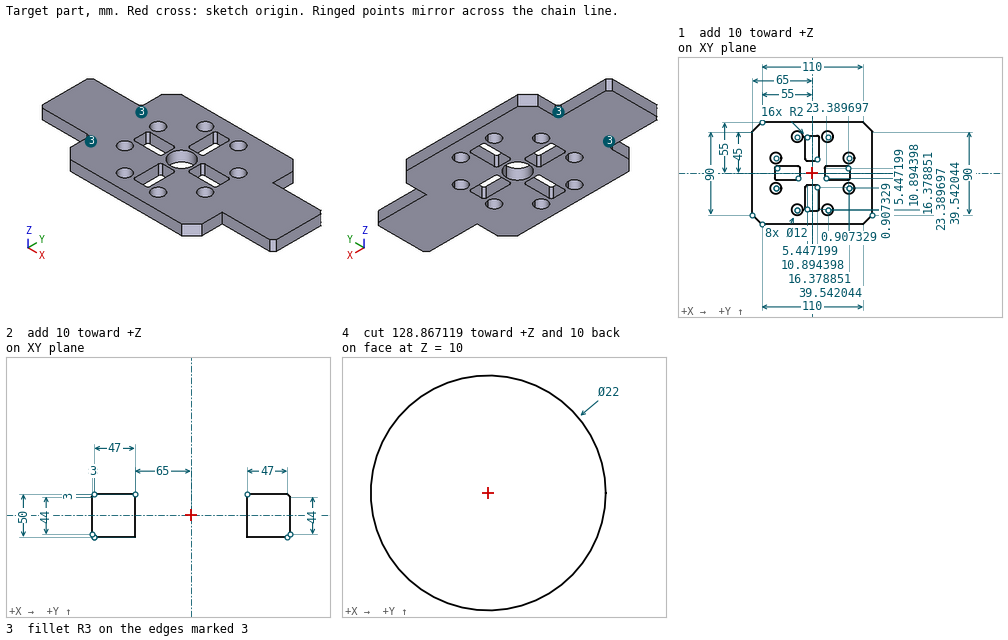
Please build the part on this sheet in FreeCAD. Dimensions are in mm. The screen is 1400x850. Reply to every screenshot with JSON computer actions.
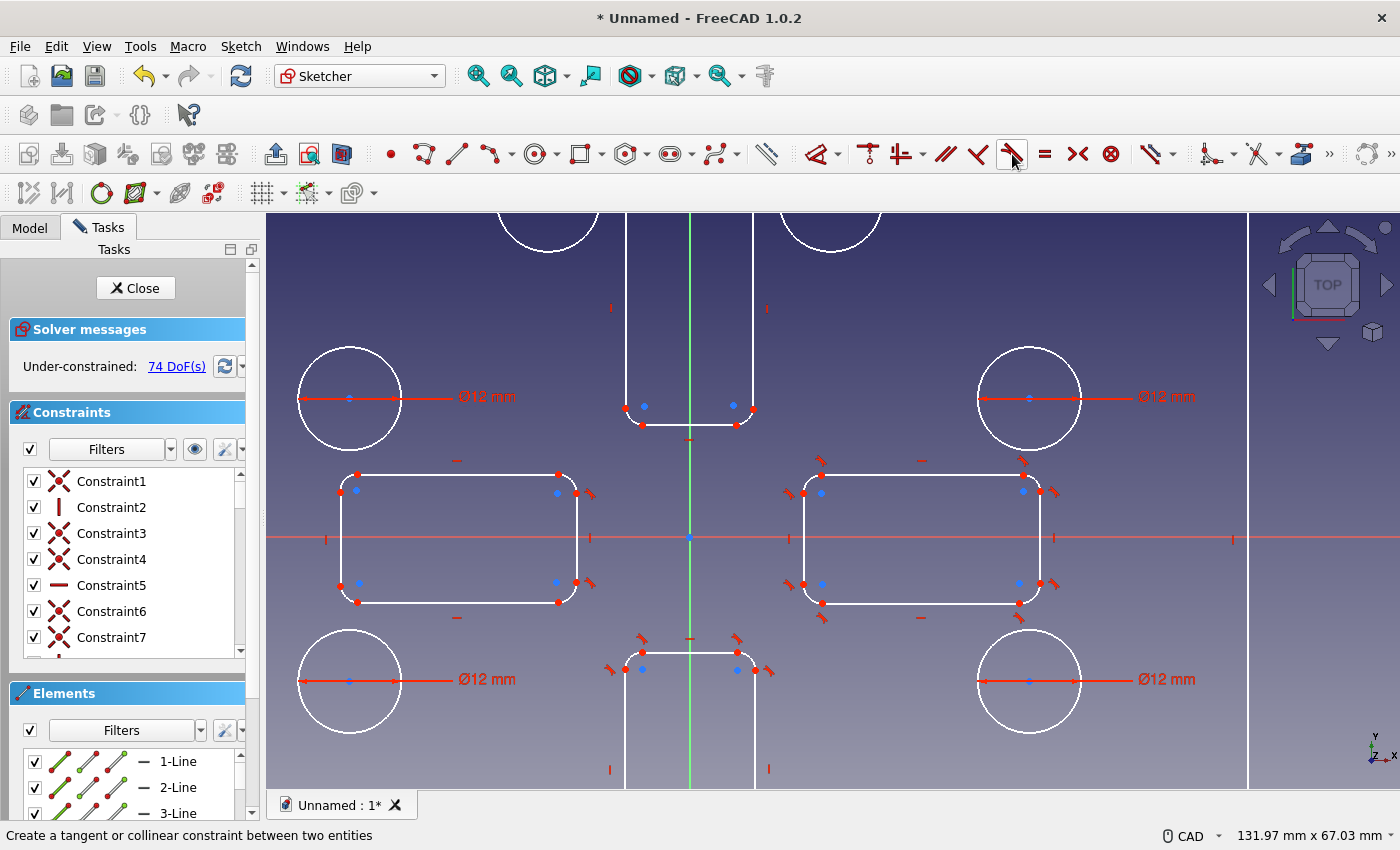
{"action": "left_click", "coordinate": [498, 603]}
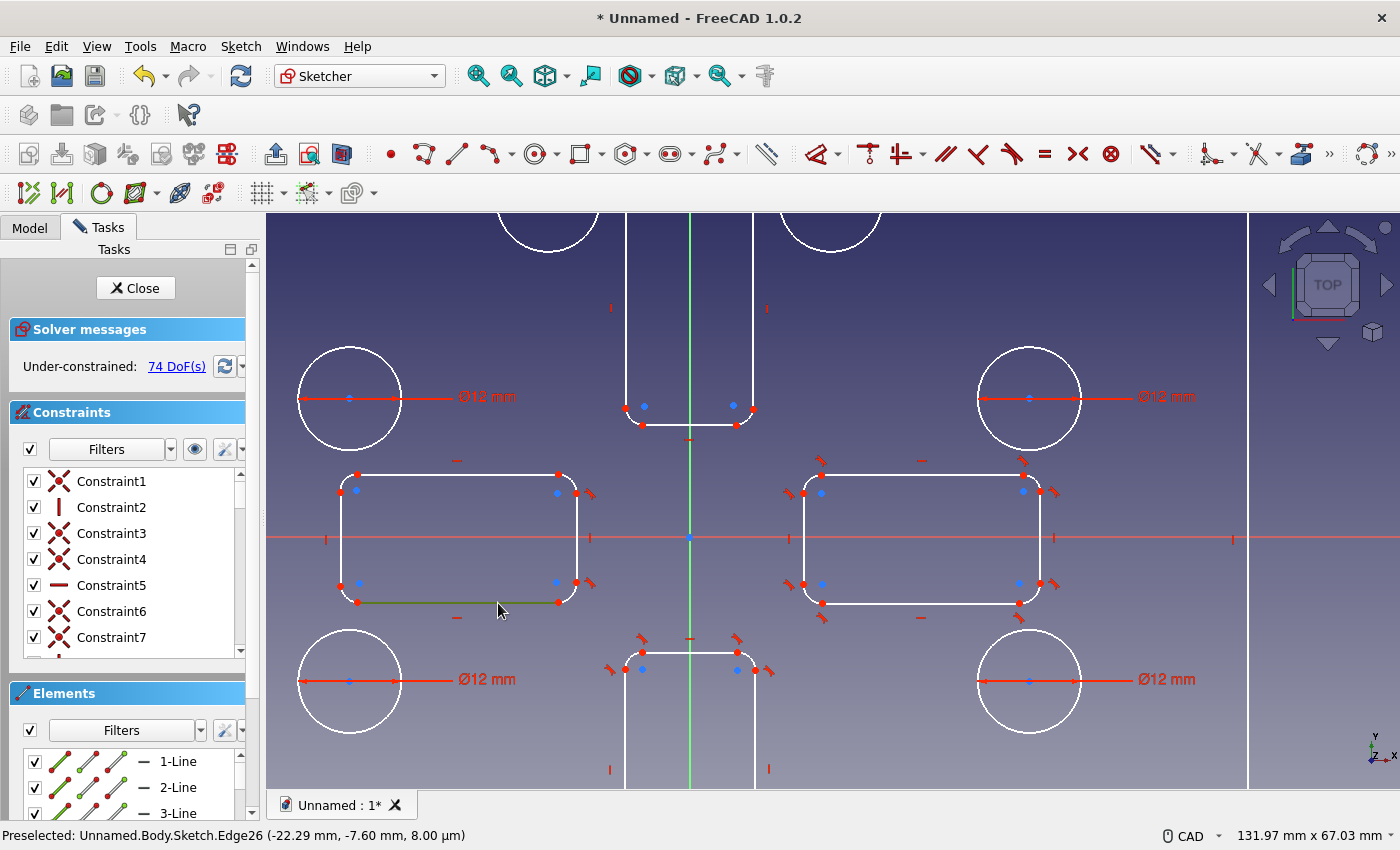
{"action": "left_click", "coordinate": [571, 596]}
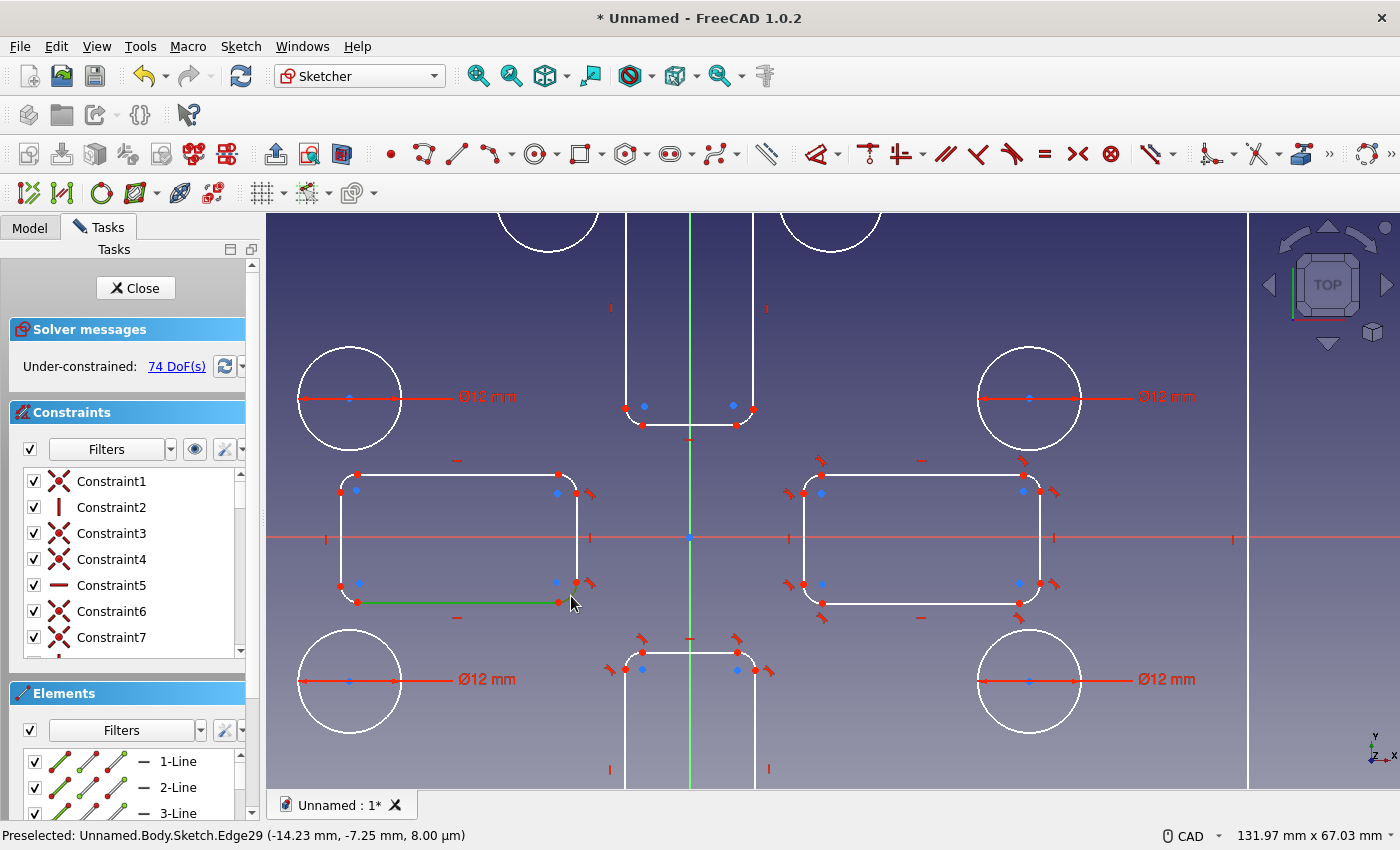
{"action": "left_click", "coordinate": [1012, 154]}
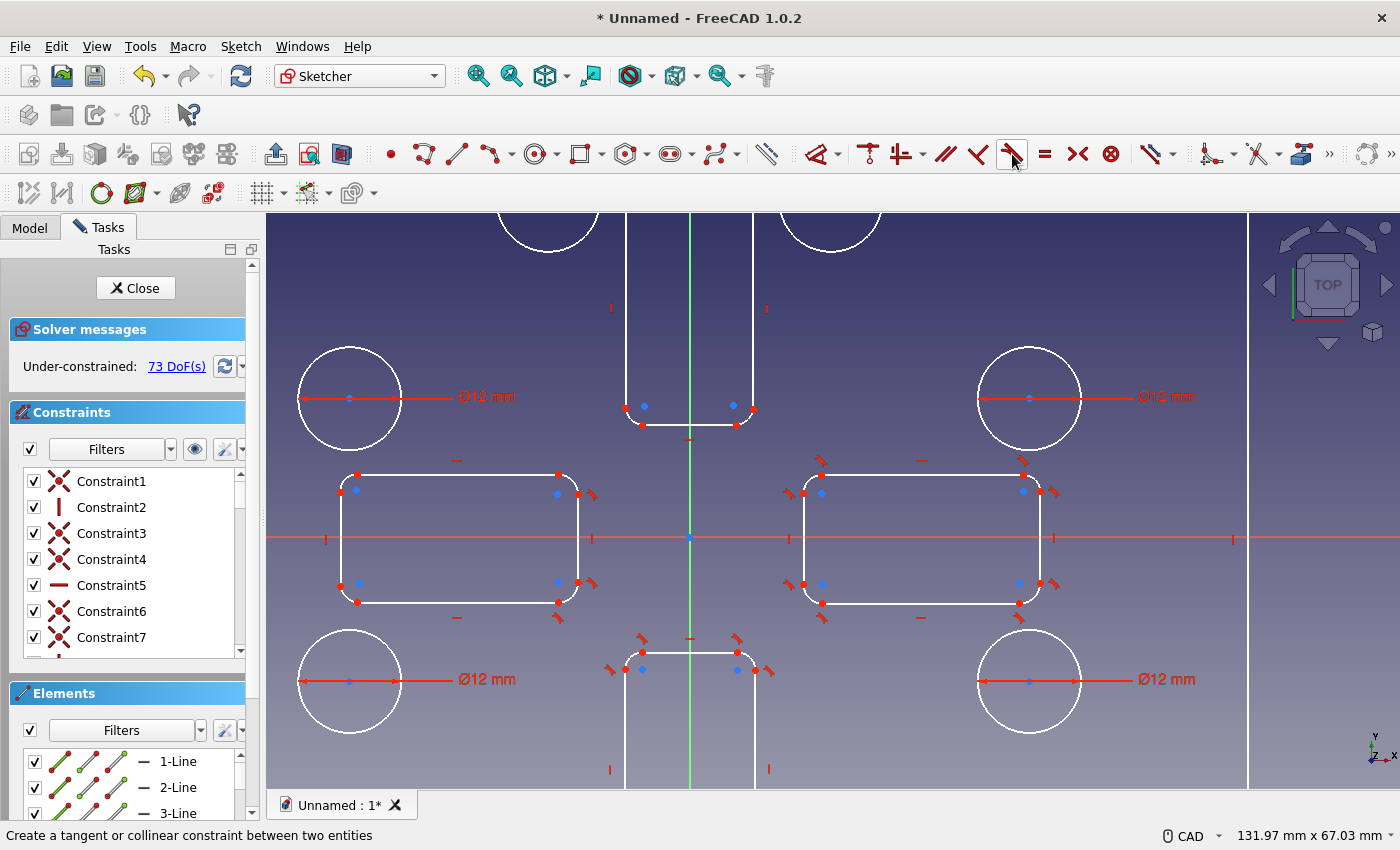
{"action": "left_click", "coordinate": [498, 603]}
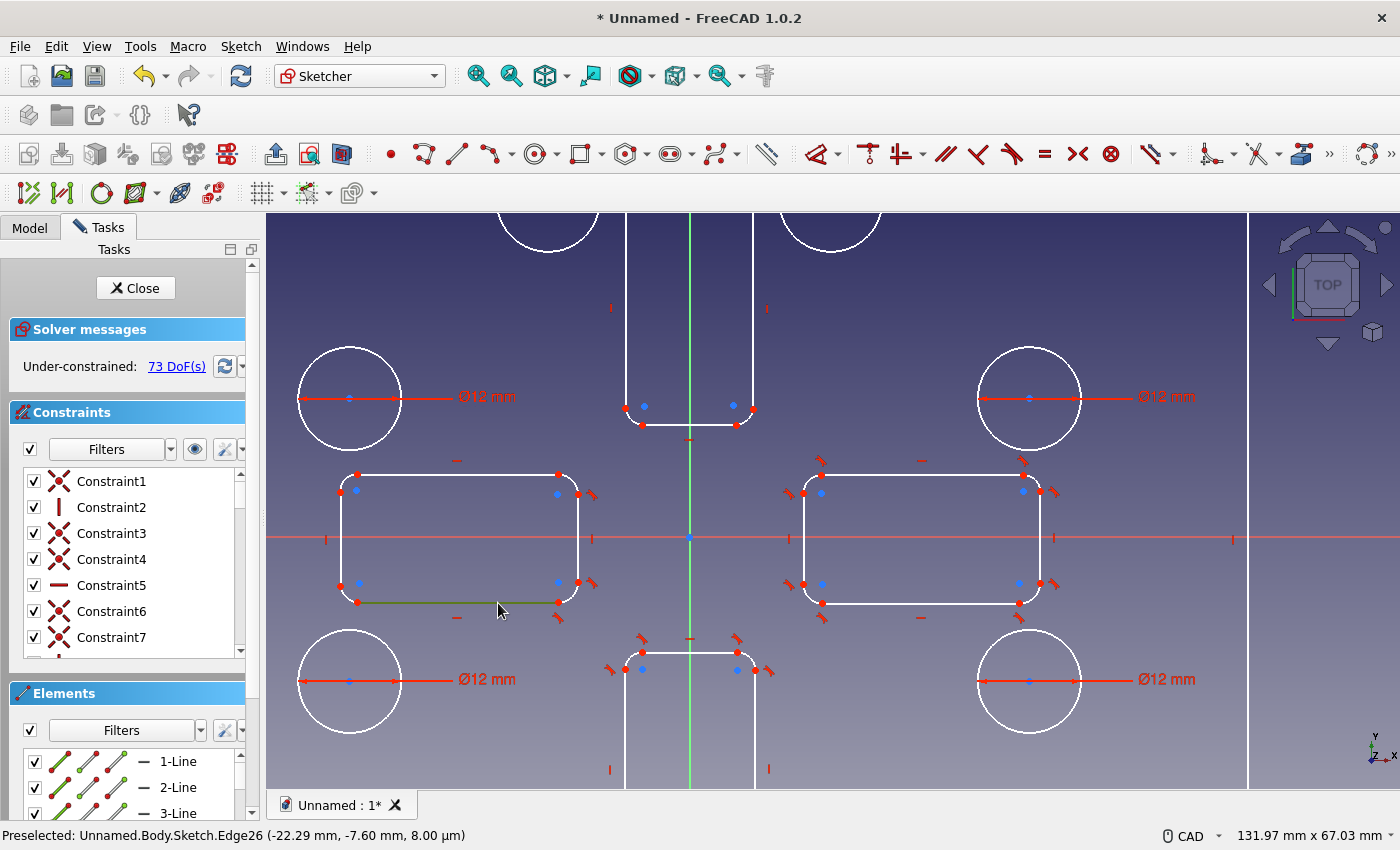
{"action": "left_click", "coordinate": [346, 597]}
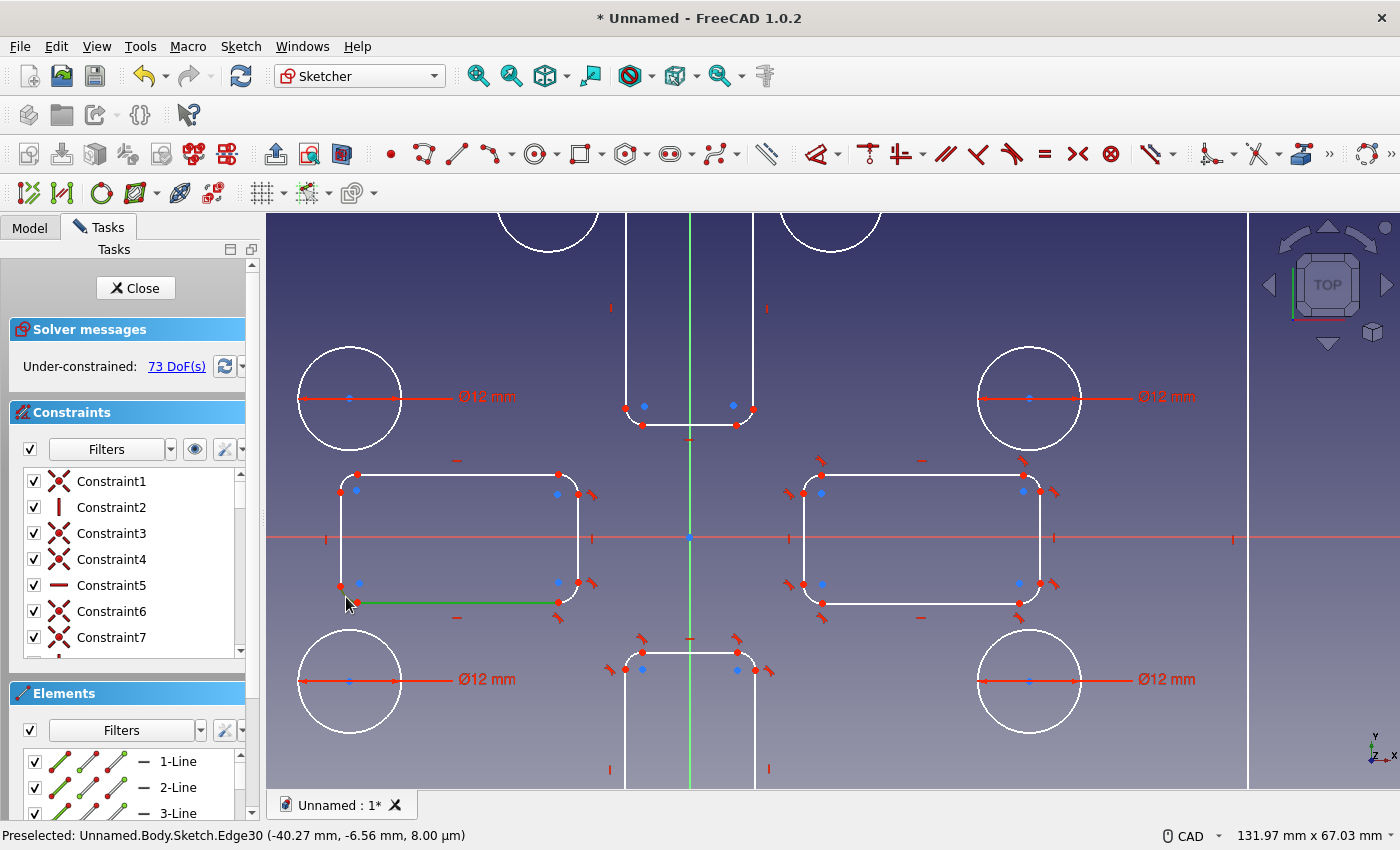
{"action": "left_click", "coordinate": [1012, 154]}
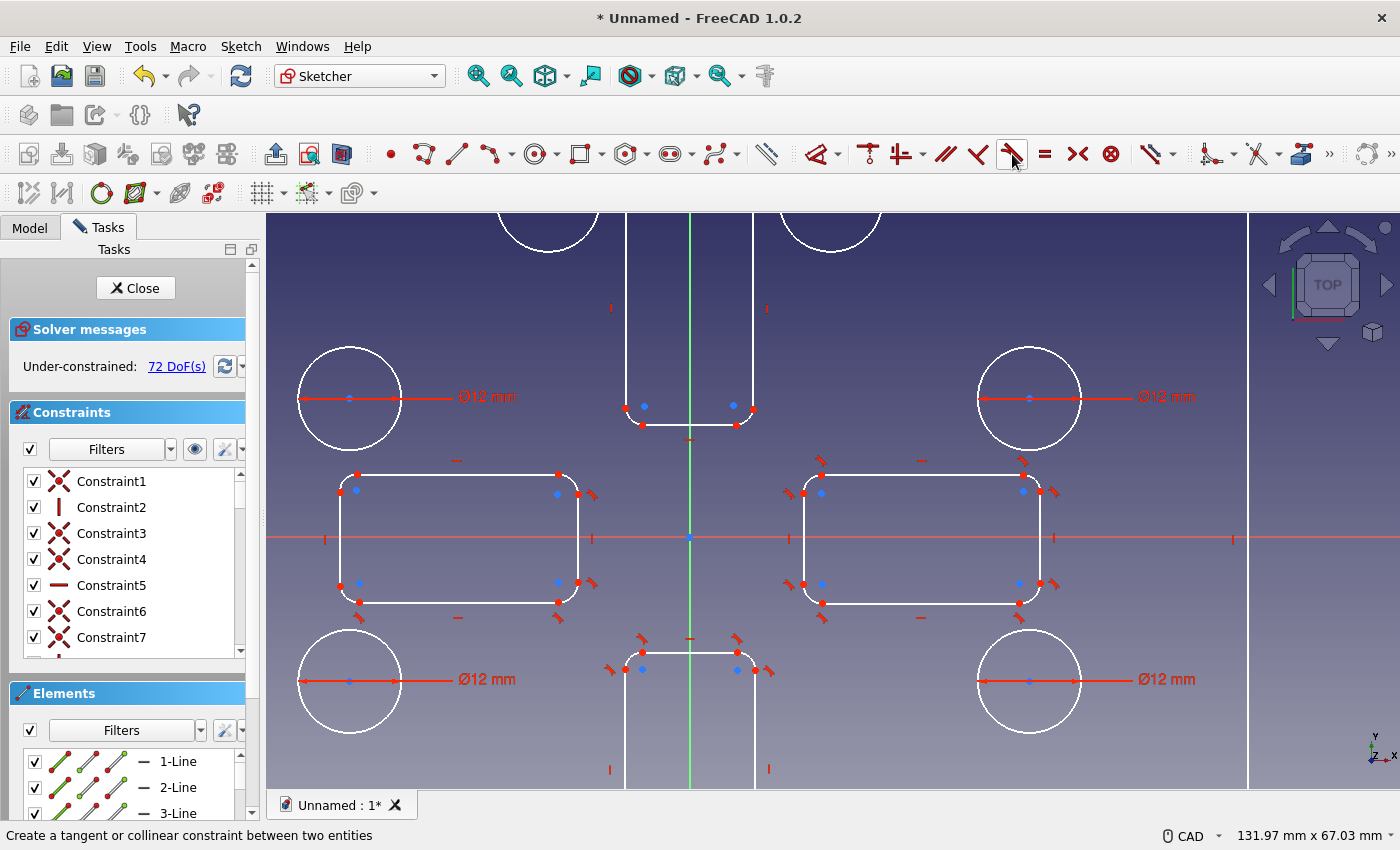
{"action": "left_click", "coordinate": [340, 558]}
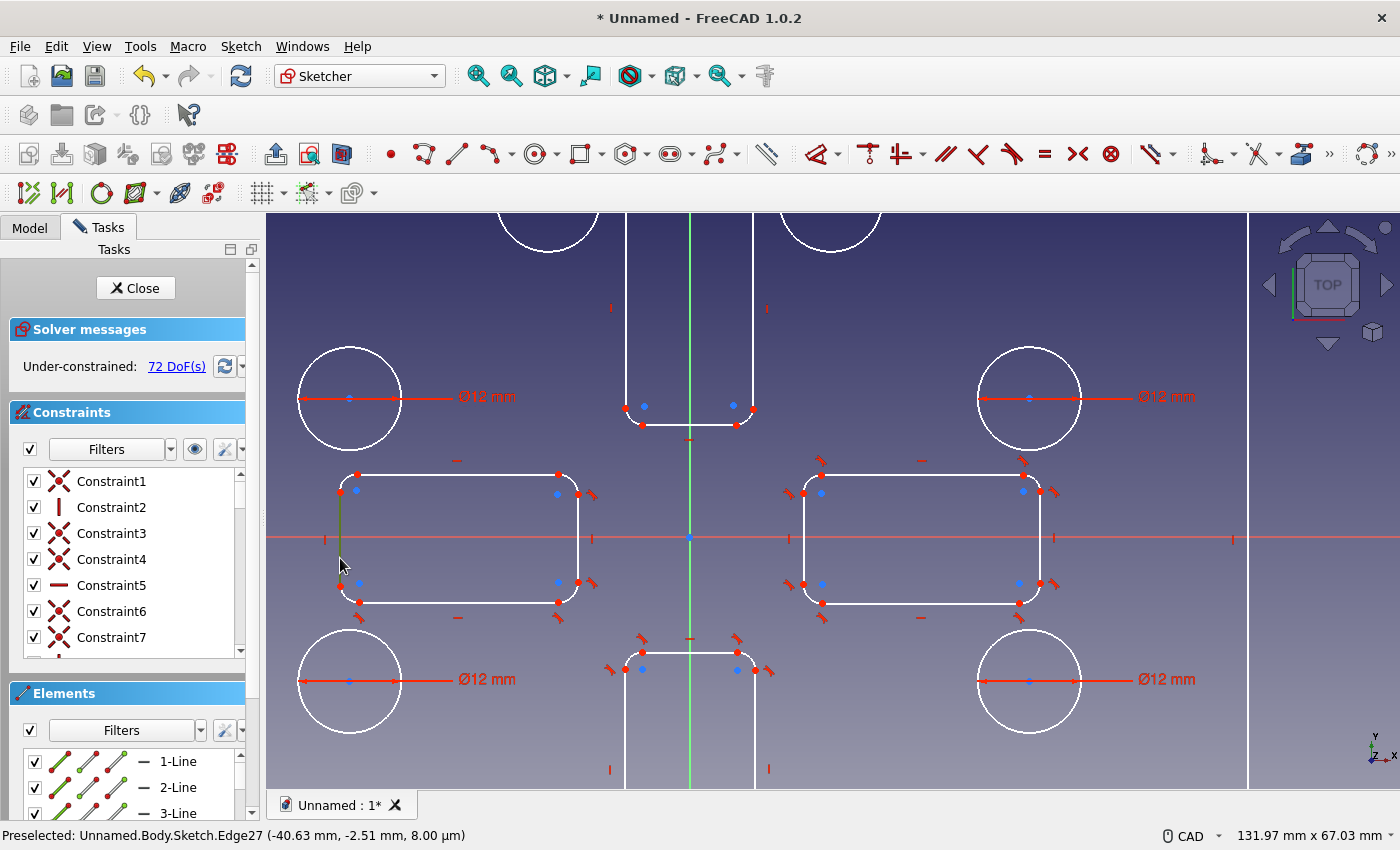
{"action": "left_click", "coordinate": [347, 598]}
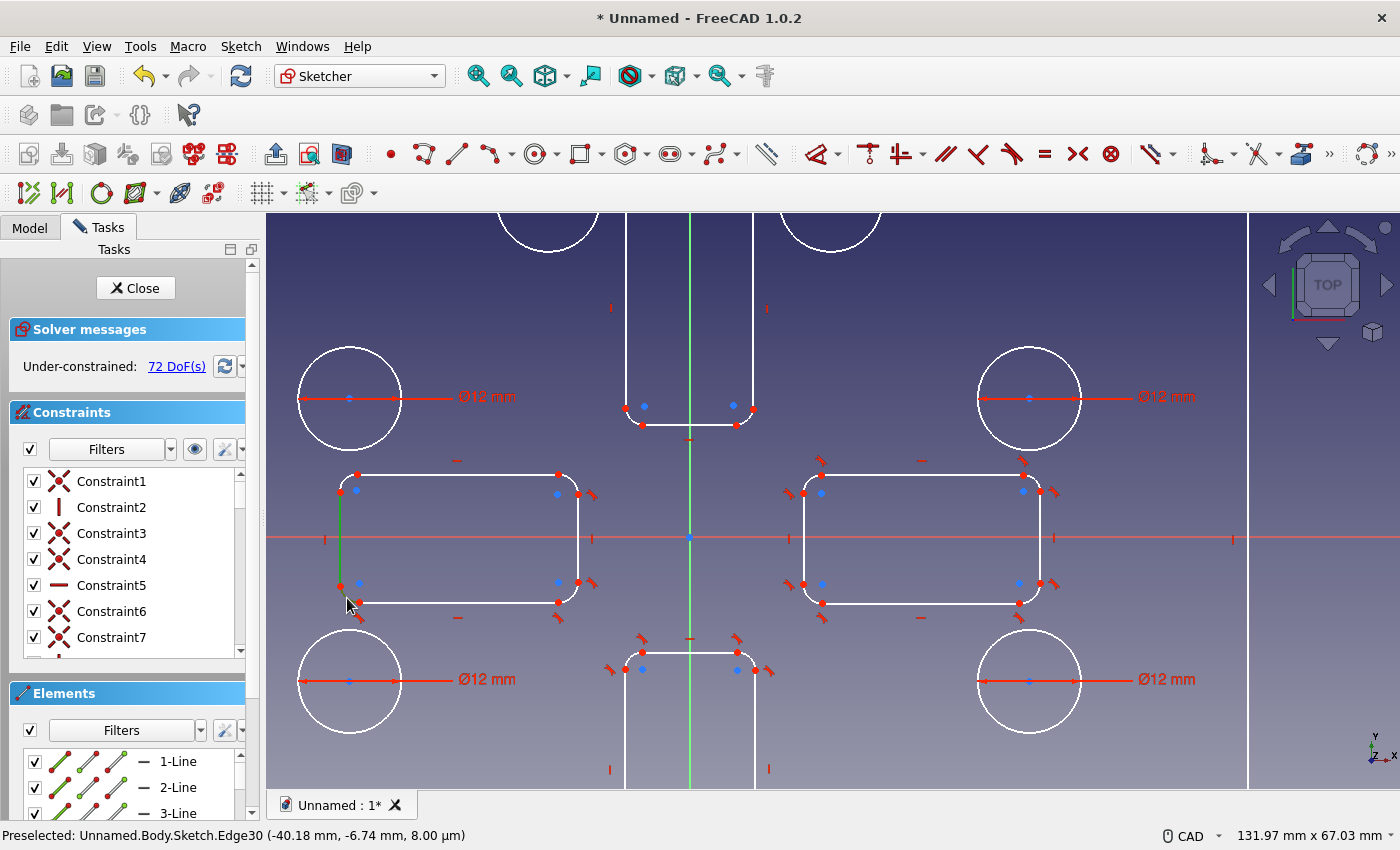
{"action": "left_click", "coordinate": [1012, 154]}